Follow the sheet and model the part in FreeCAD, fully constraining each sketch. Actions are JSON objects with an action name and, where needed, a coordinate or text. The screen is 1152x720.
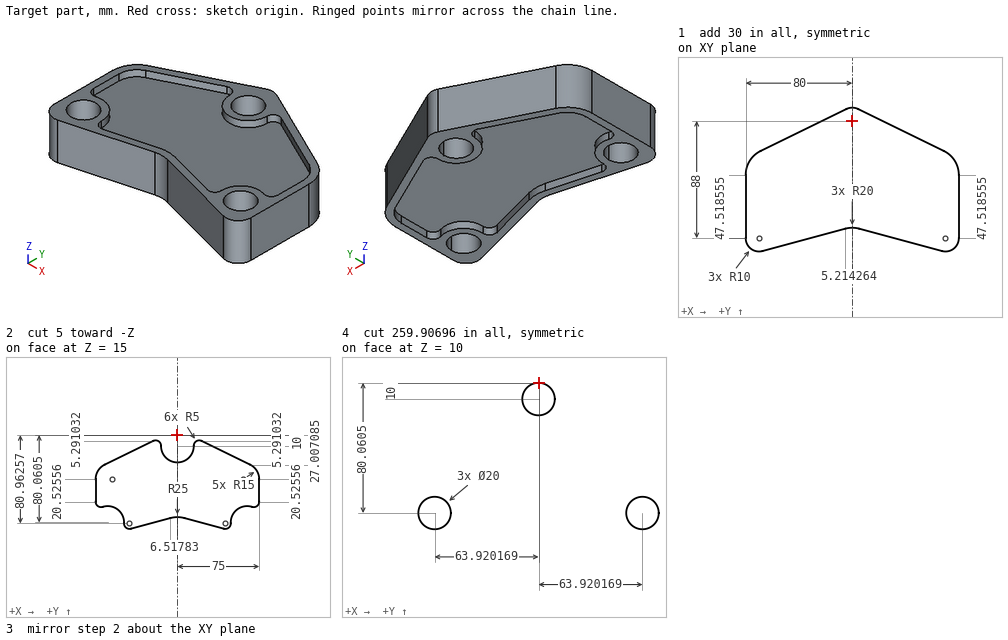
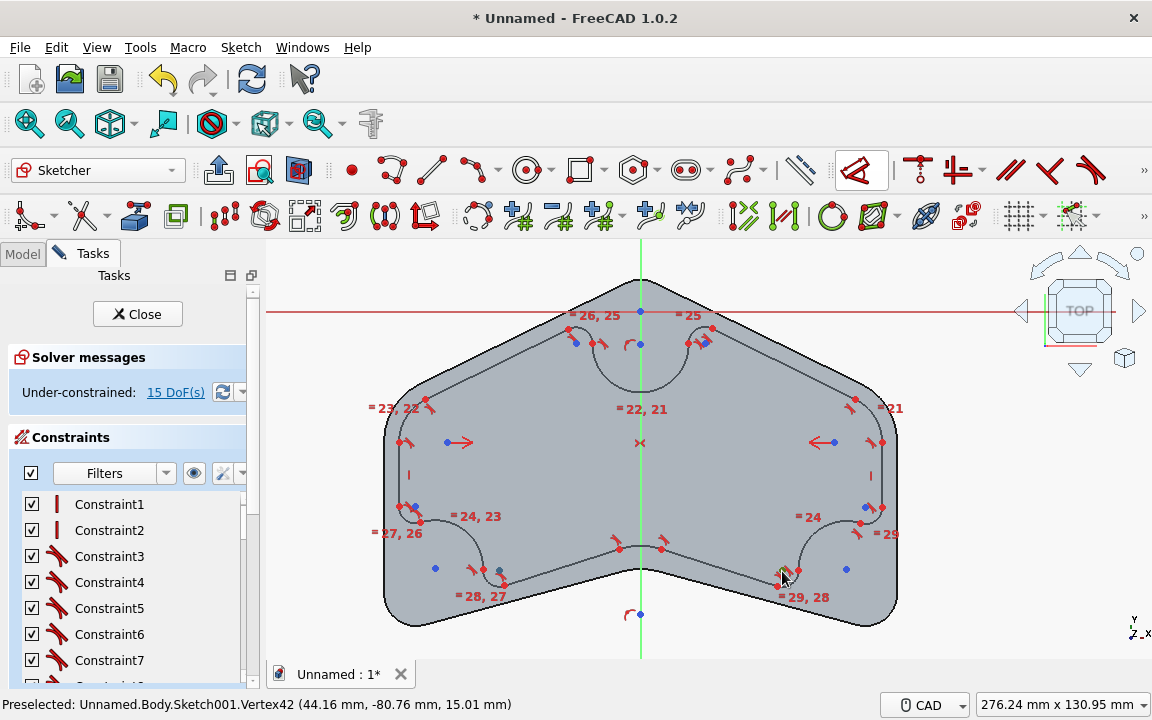
{"action": "left_click", "coordinate": [641, 605]}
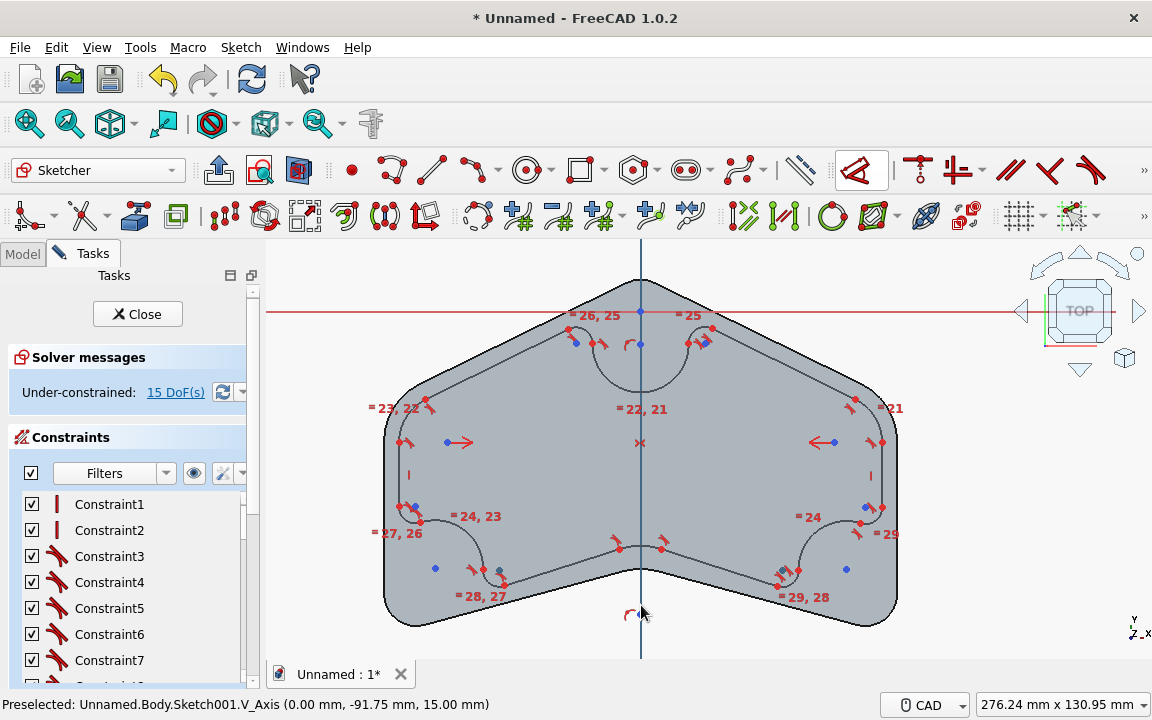
{"action": "key", "text": "s"}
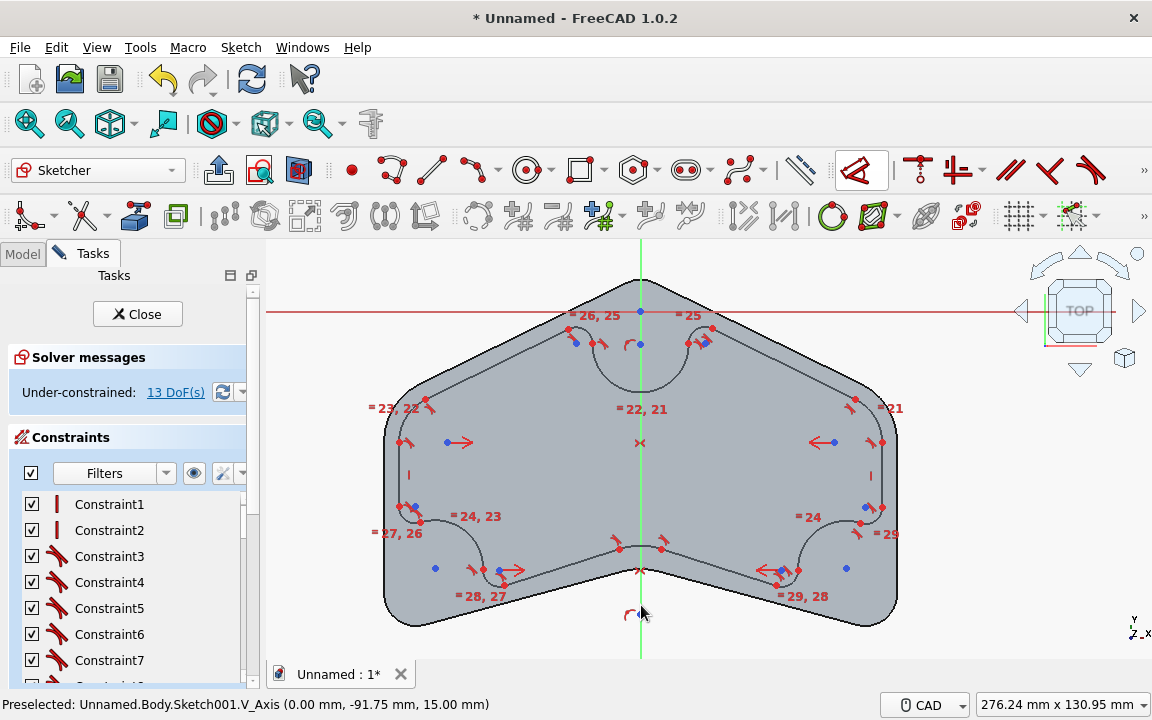
{"action": "left_click", "coordinate": [879, 427]}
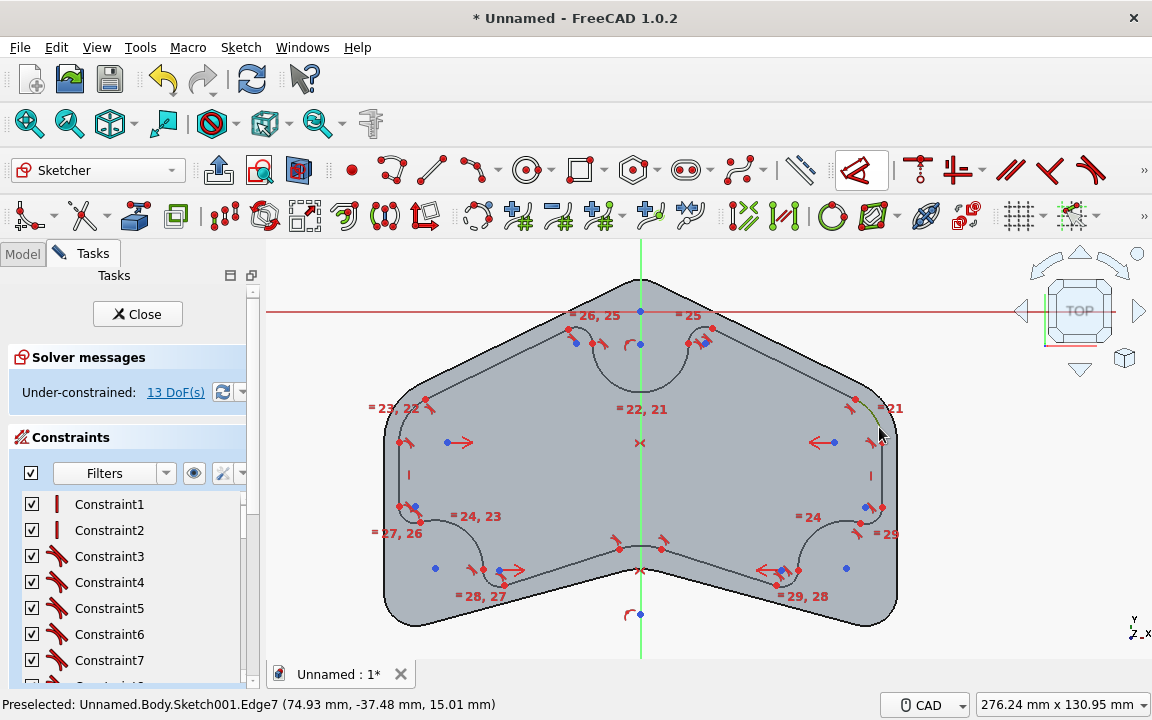
{"action": "left_click", "coordinate": [882, 170]}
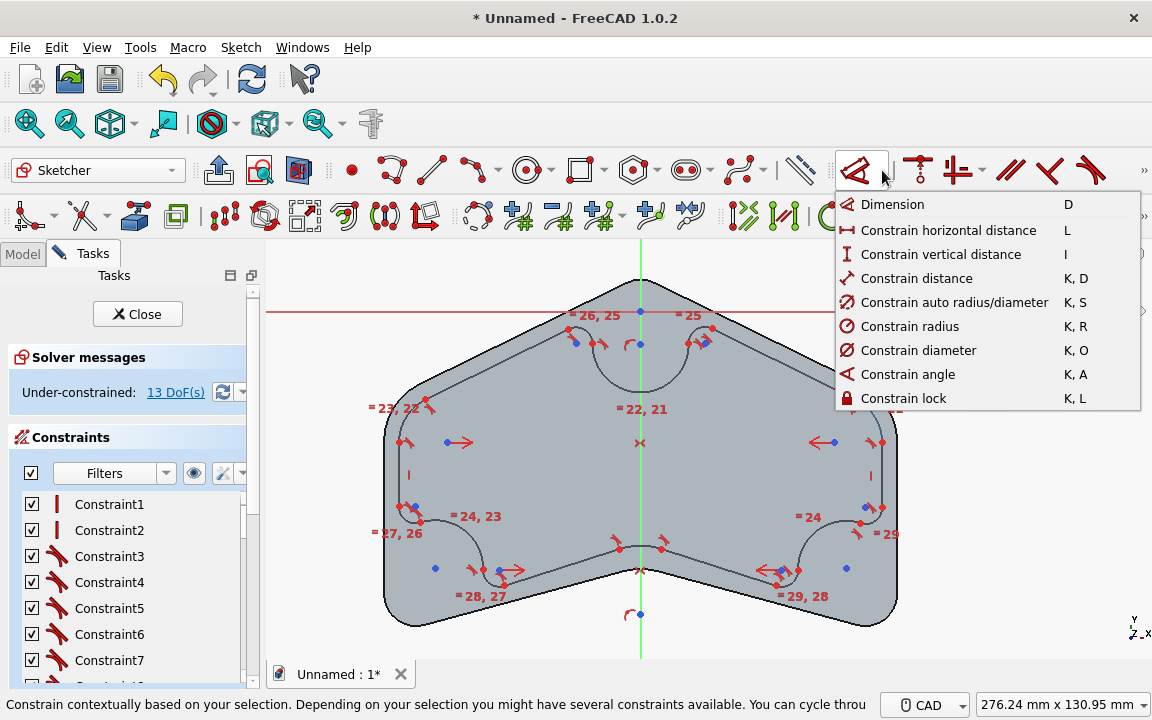
{"action": "left_click", "coordinate": [988, 326]}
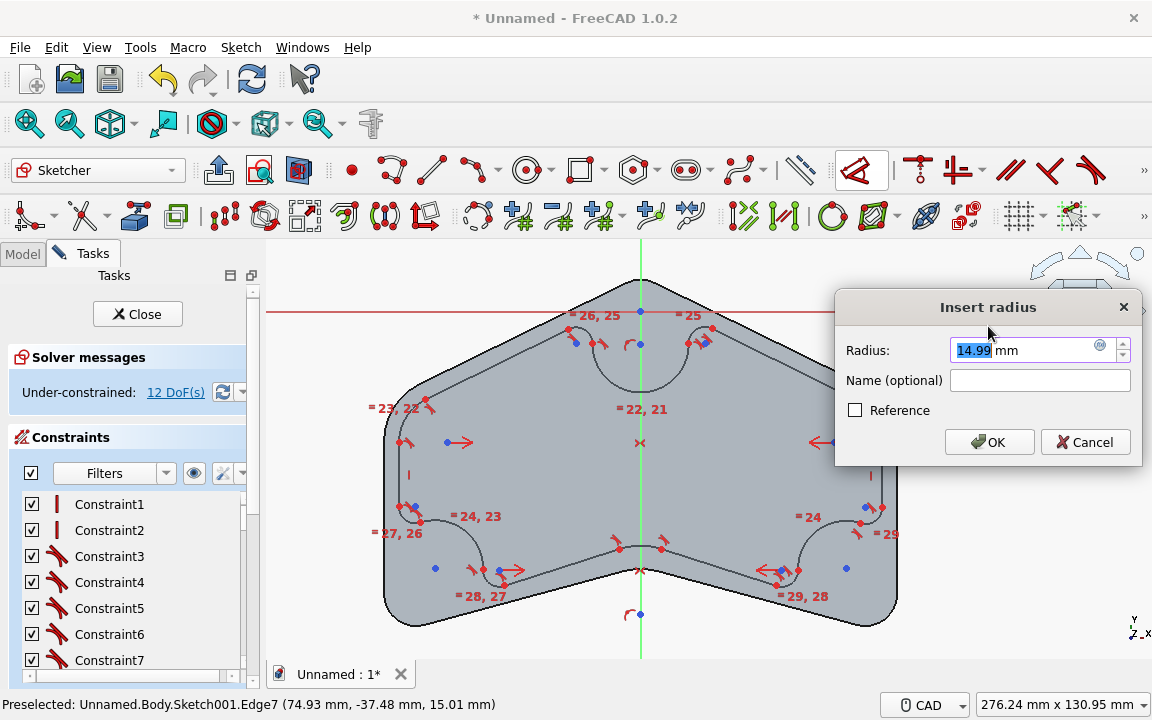
{"action": "type", "text": "15"}
{"action": "key", "text": "Return"}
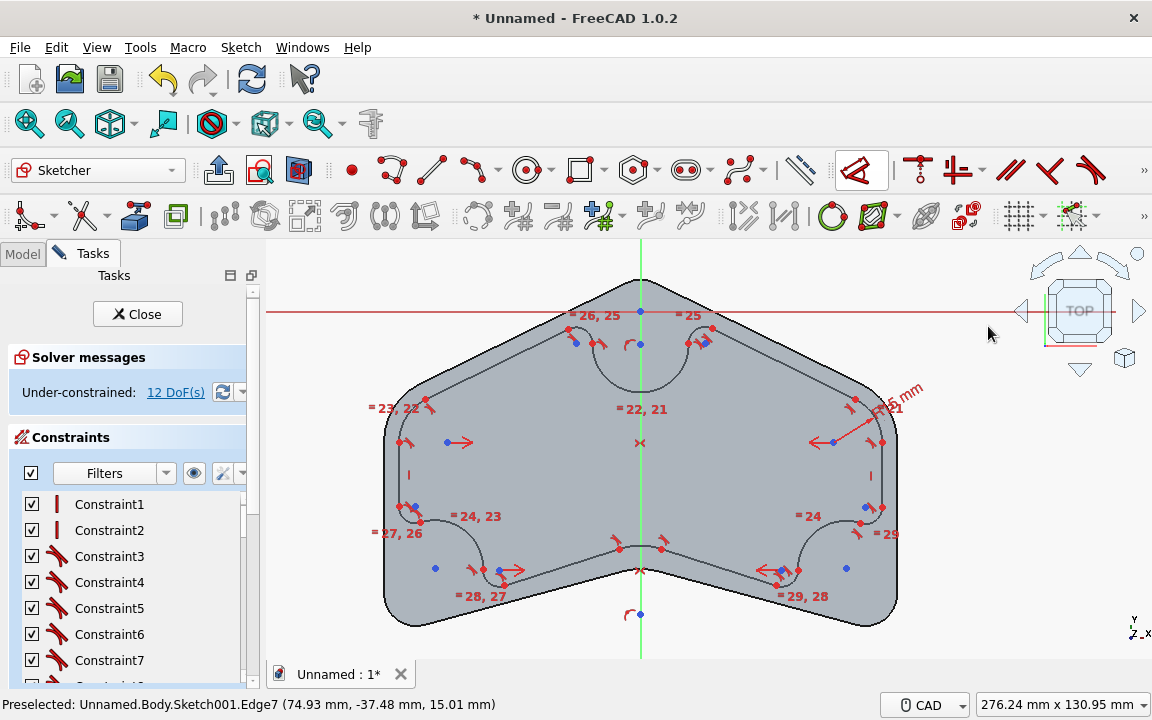
{"action": "scroll", "coordinate": [703, 327], "scroll_direction": "up", "scroll_amount": 5}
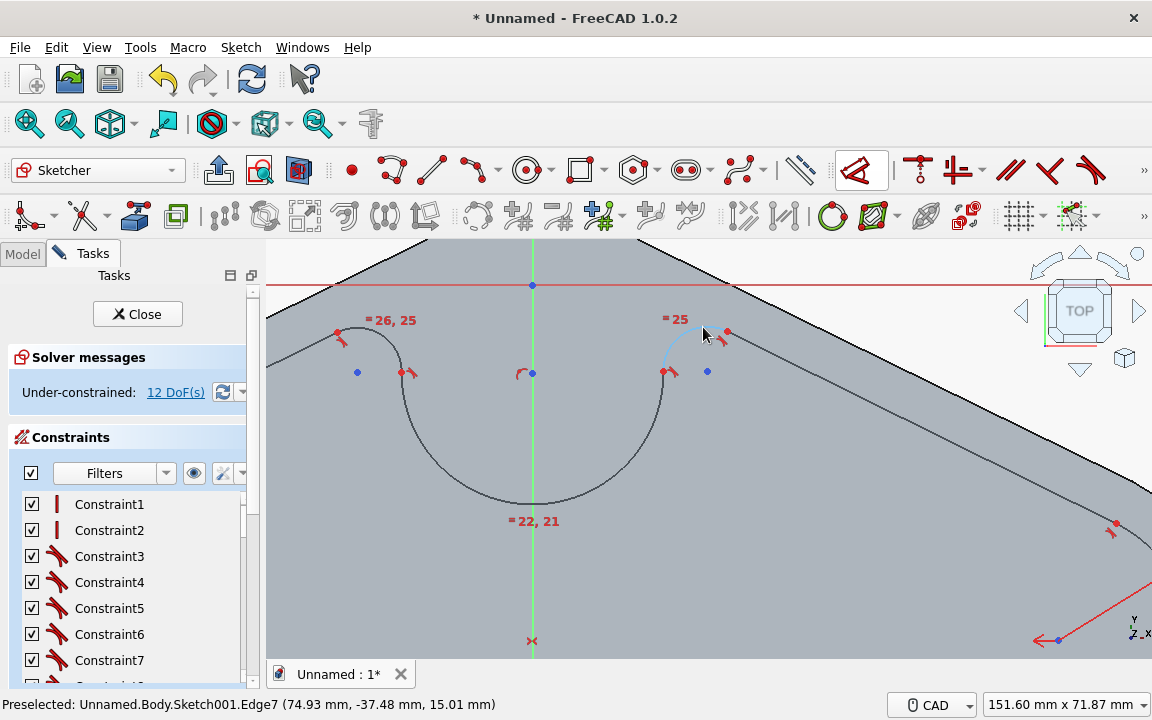
{"action": "left_click", "coordinate": [701, 327]}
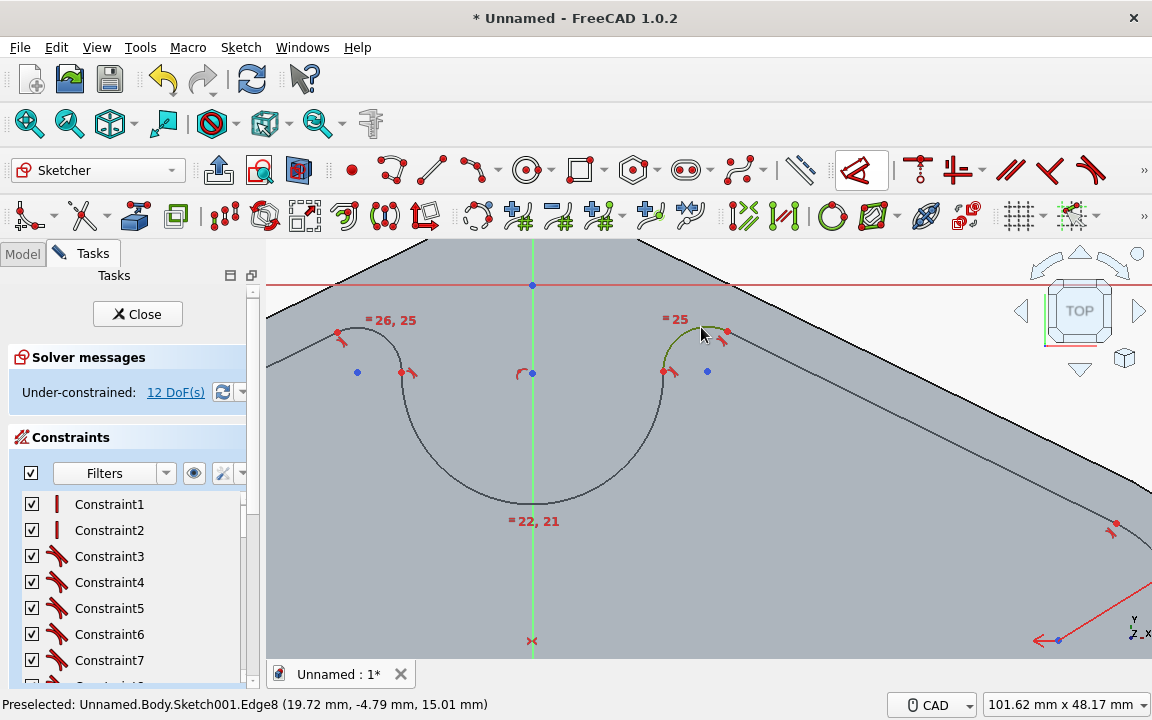
{"action": "left_click", "coordinate": [882, 170]}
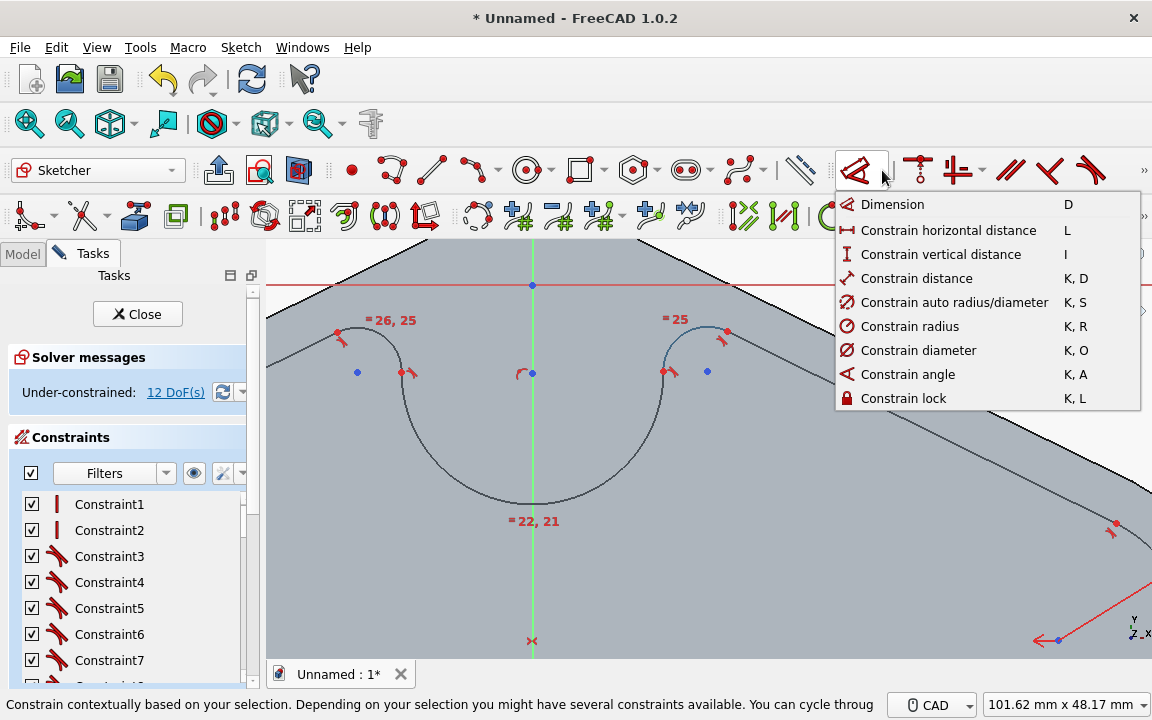
{"action": "left_click", "coordinate": [988, 326]}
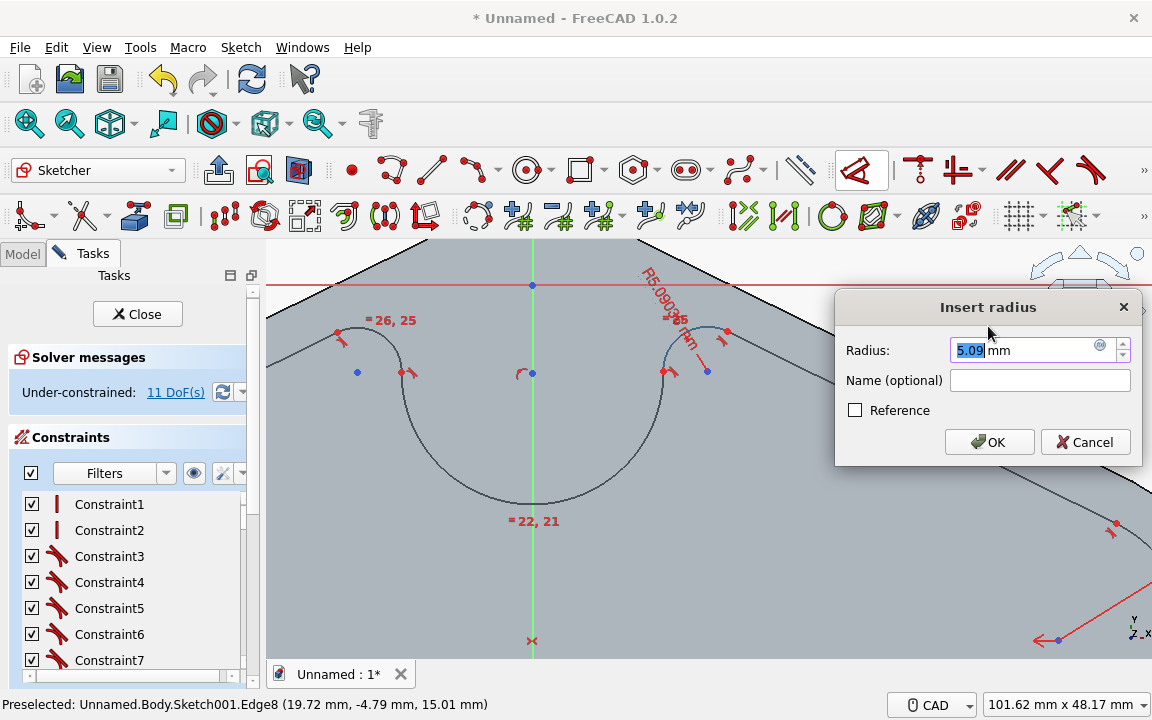
{"action": "type", "text": "5"}
{"action": "key", "text": "Return"}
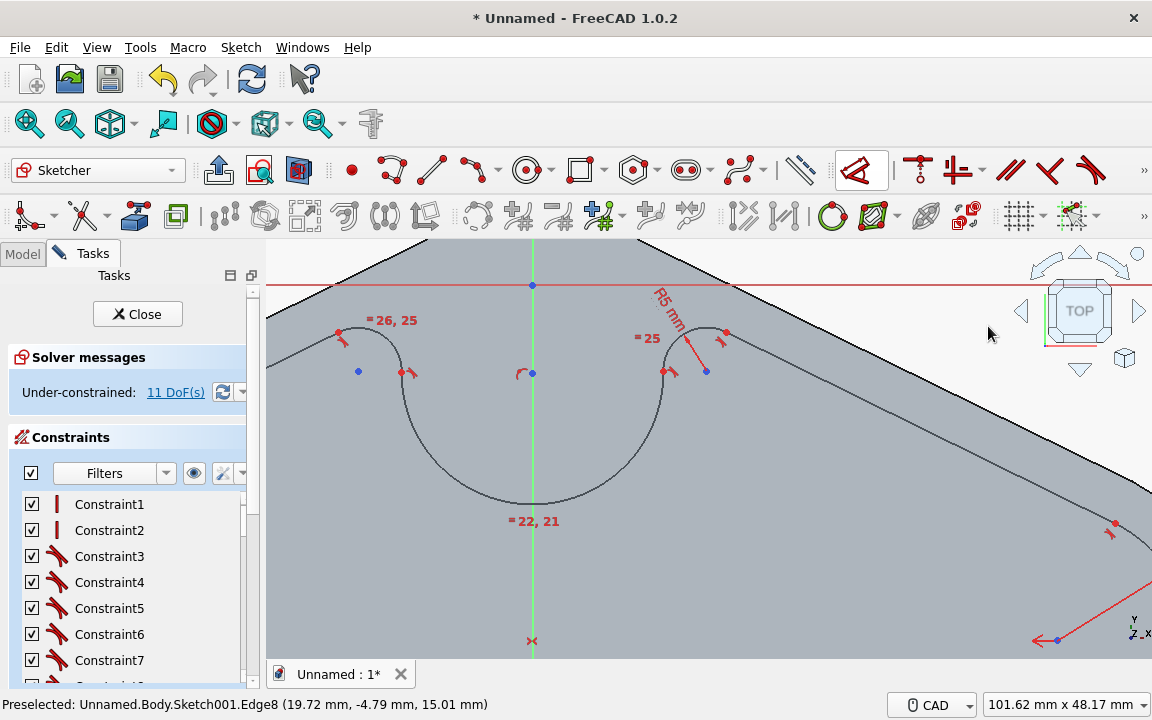
{"action": "scroll", "coordinate": [703, 327], "scroll_direction": "down", "scroll_amount": 5}